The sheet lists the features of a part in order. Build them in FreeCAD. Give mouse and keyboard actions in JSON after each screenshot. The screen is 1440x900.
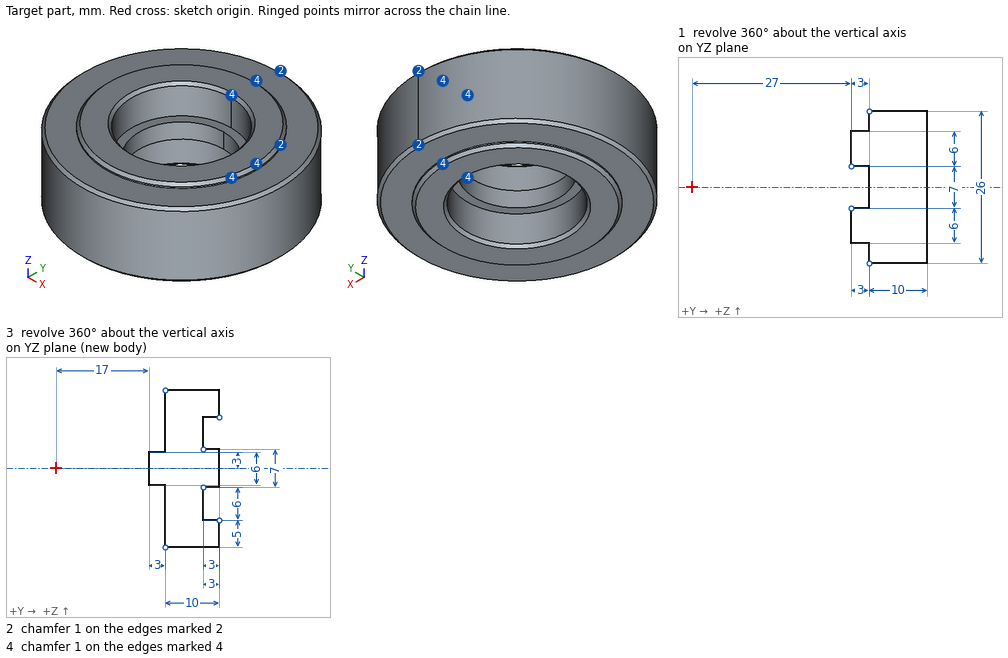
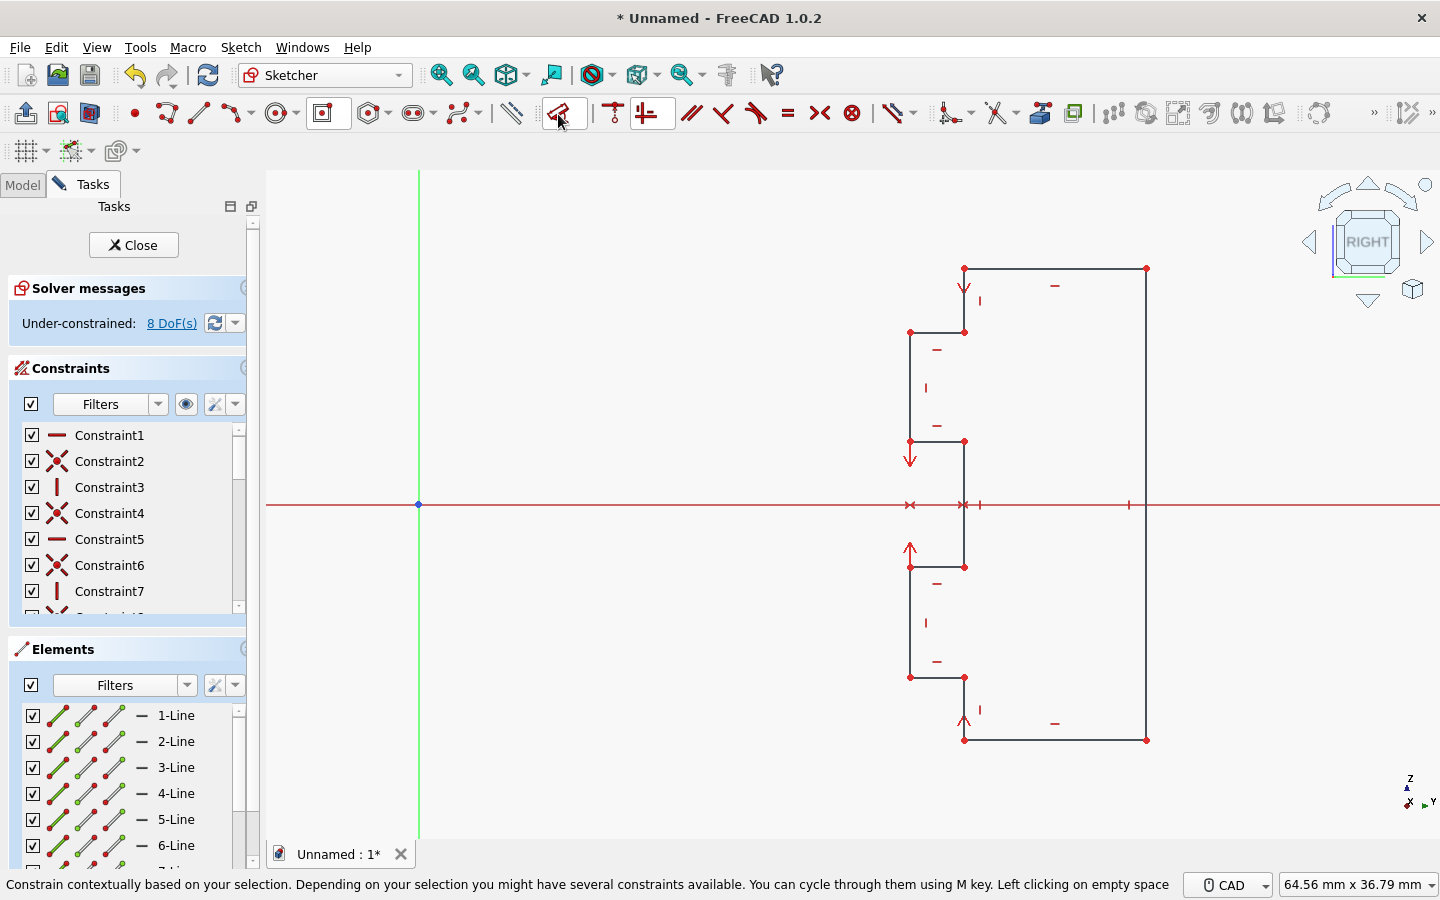
{"action": "left_click", "coordinate": [926, 442]}
{"action": "left_click", "coordinate": [937, 408]}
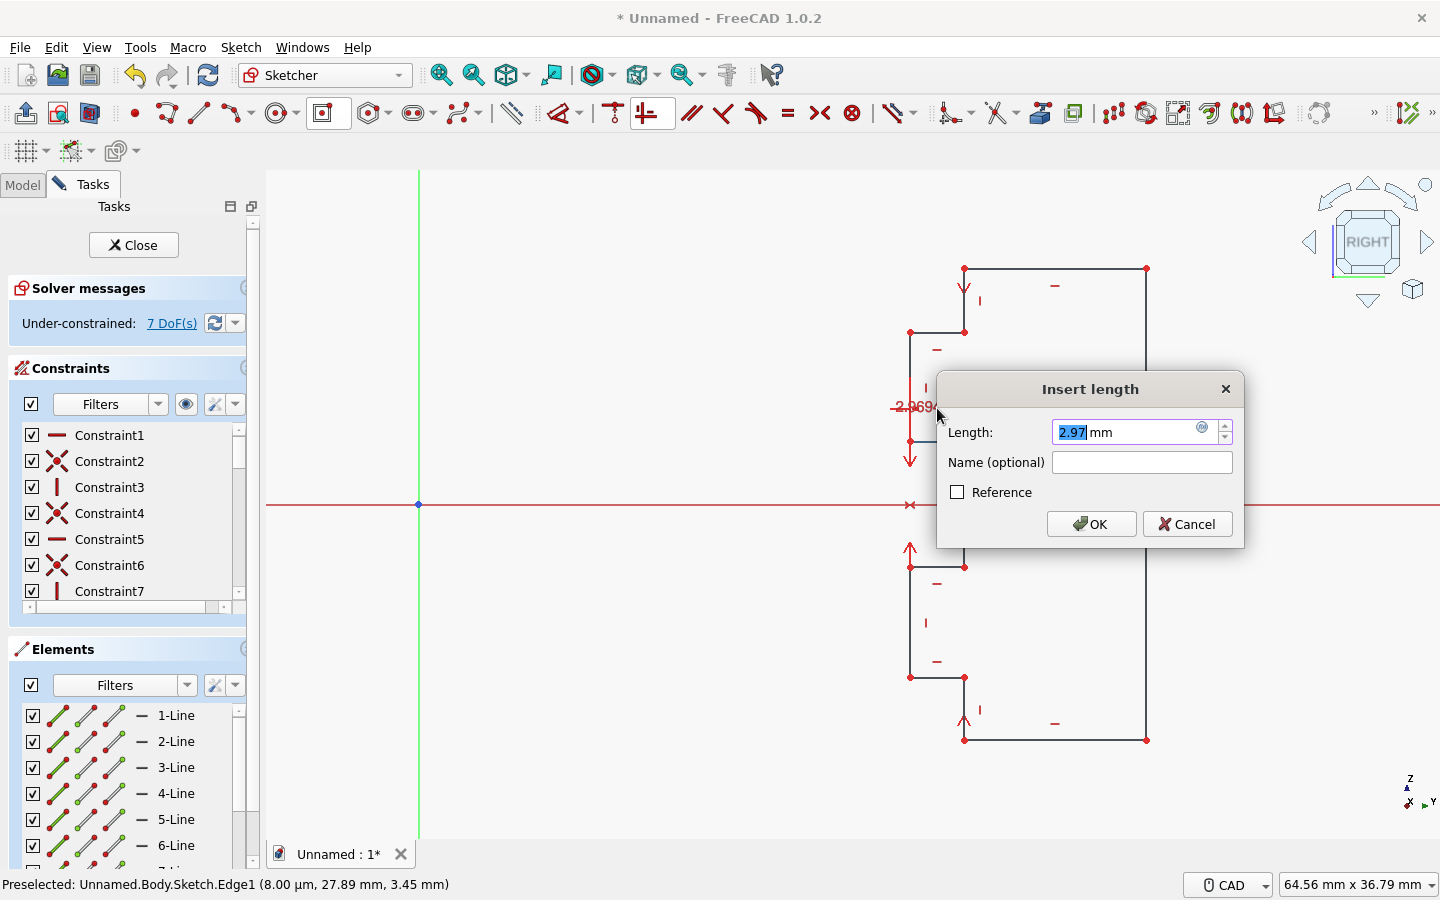
{"action": "type", "text": "3"}
{"action": "key", "text": "Return"}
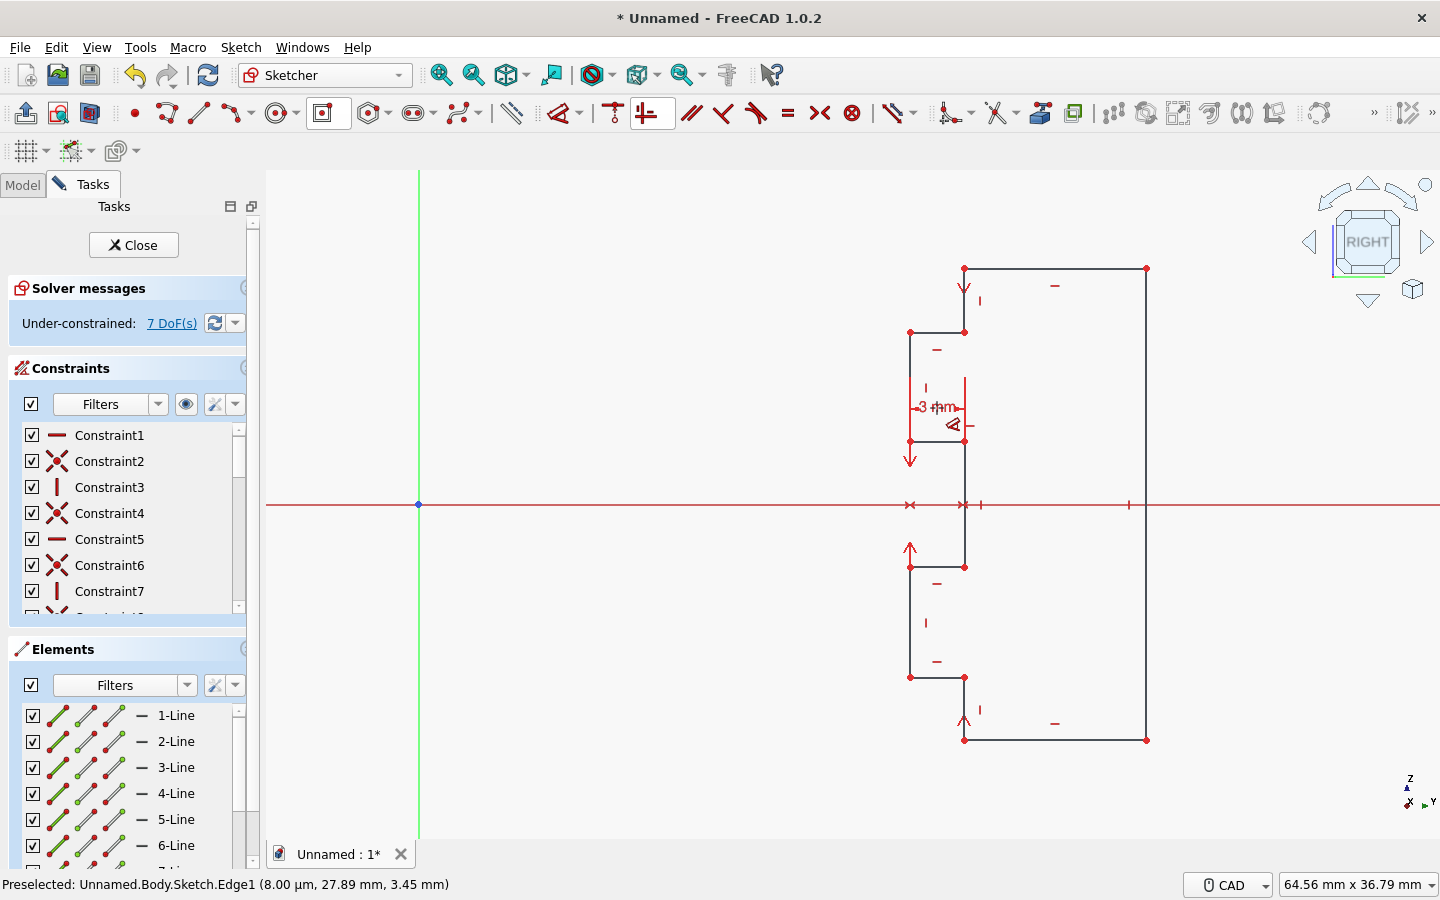
{"action": "left_click", "coordinate": [965, 479]}
{"action": "left_click", "coordinate": [999, 476]}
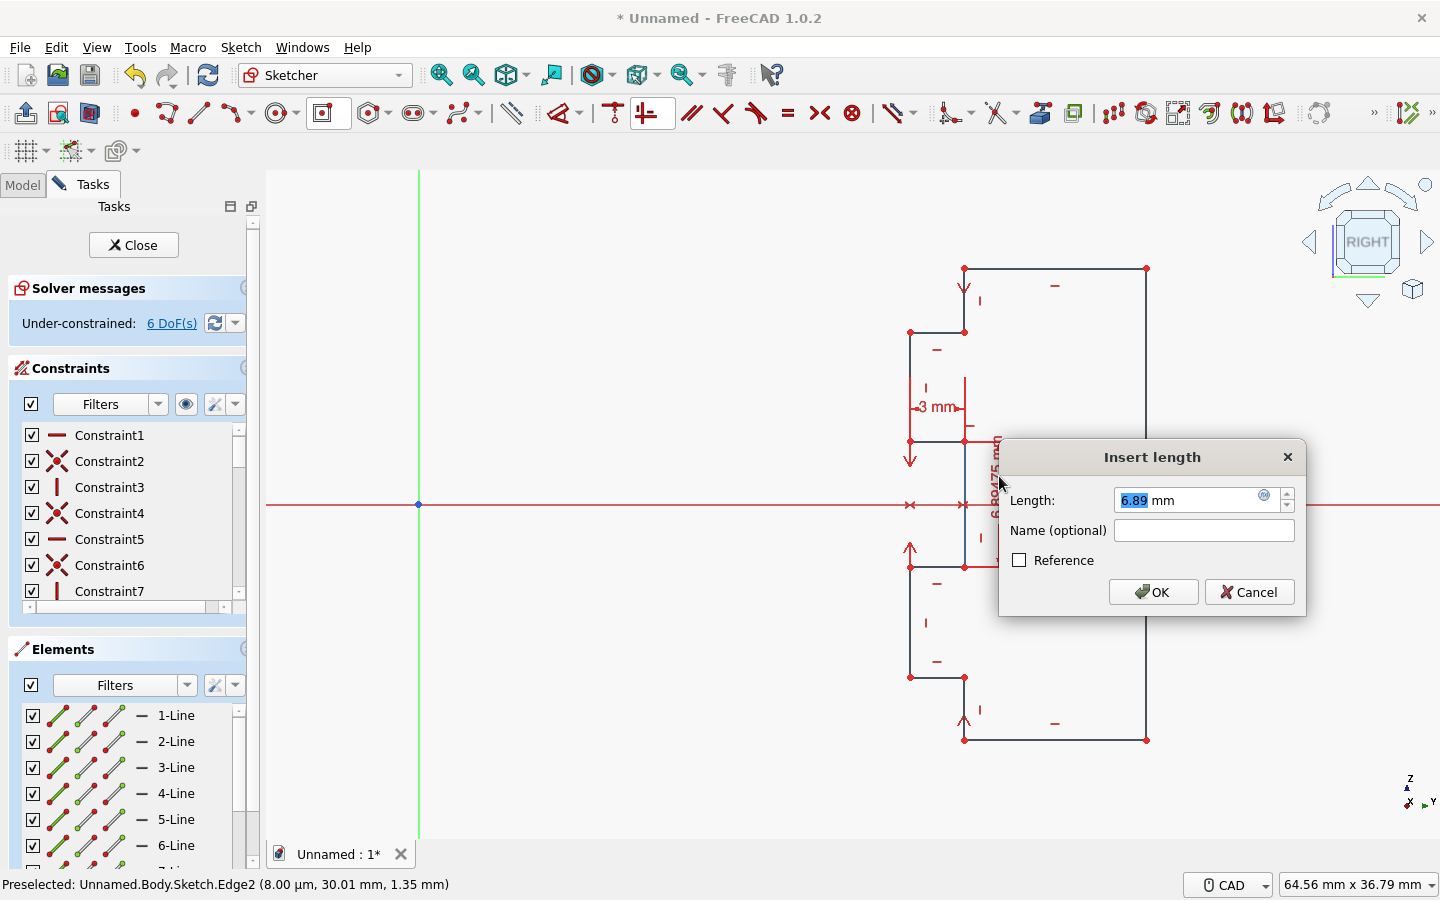
{"action": "type", "text": "7"}
{"action": "key", "text": "Return"}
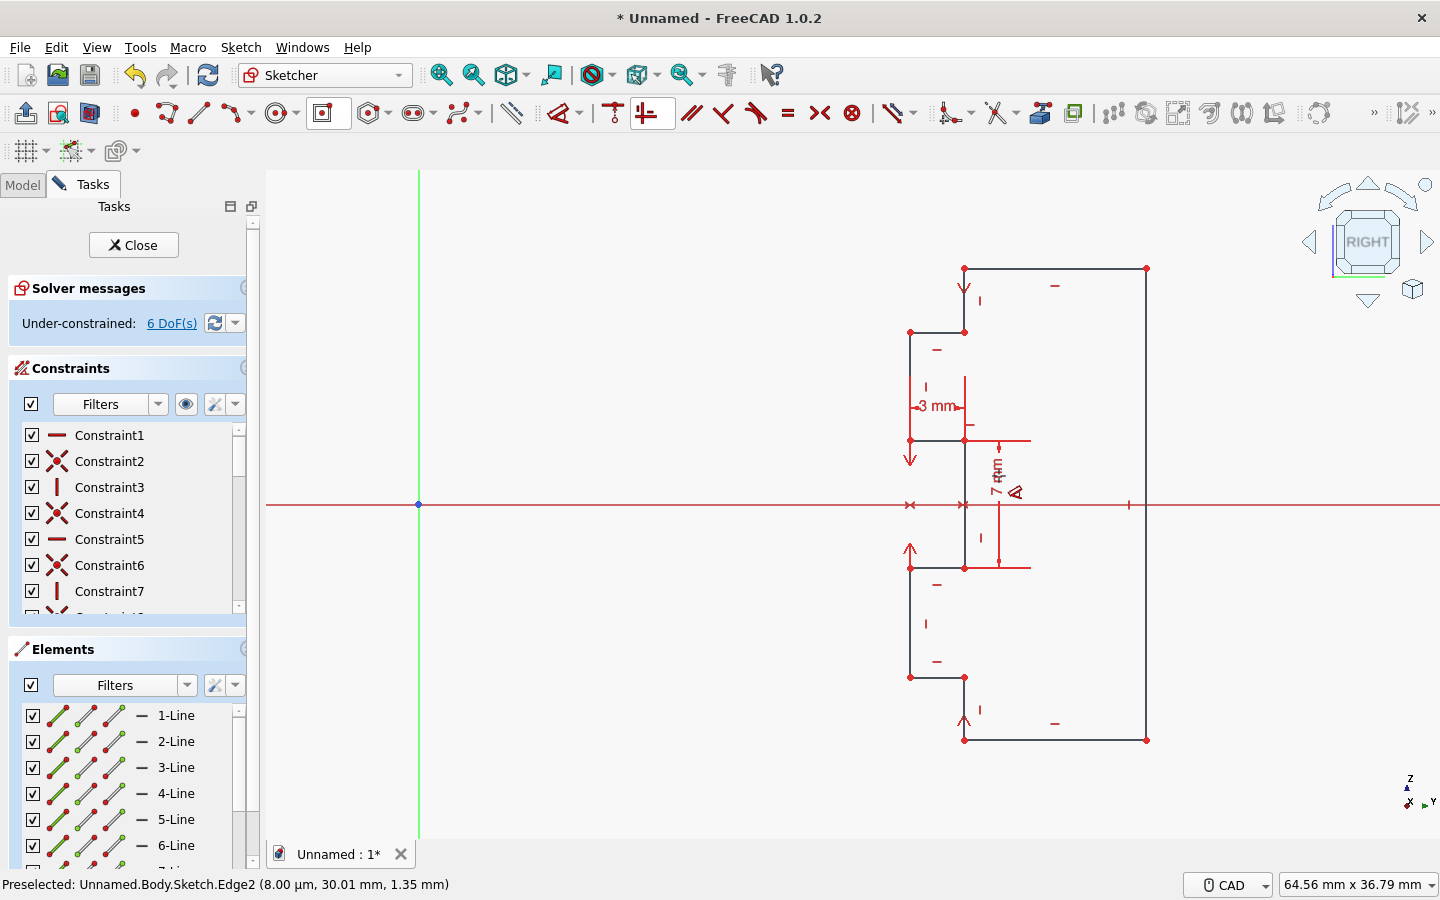
{"action": "left_click", "coordinate": [910, 601]}
{"action": "left_click", "coordinate": [944, 623]}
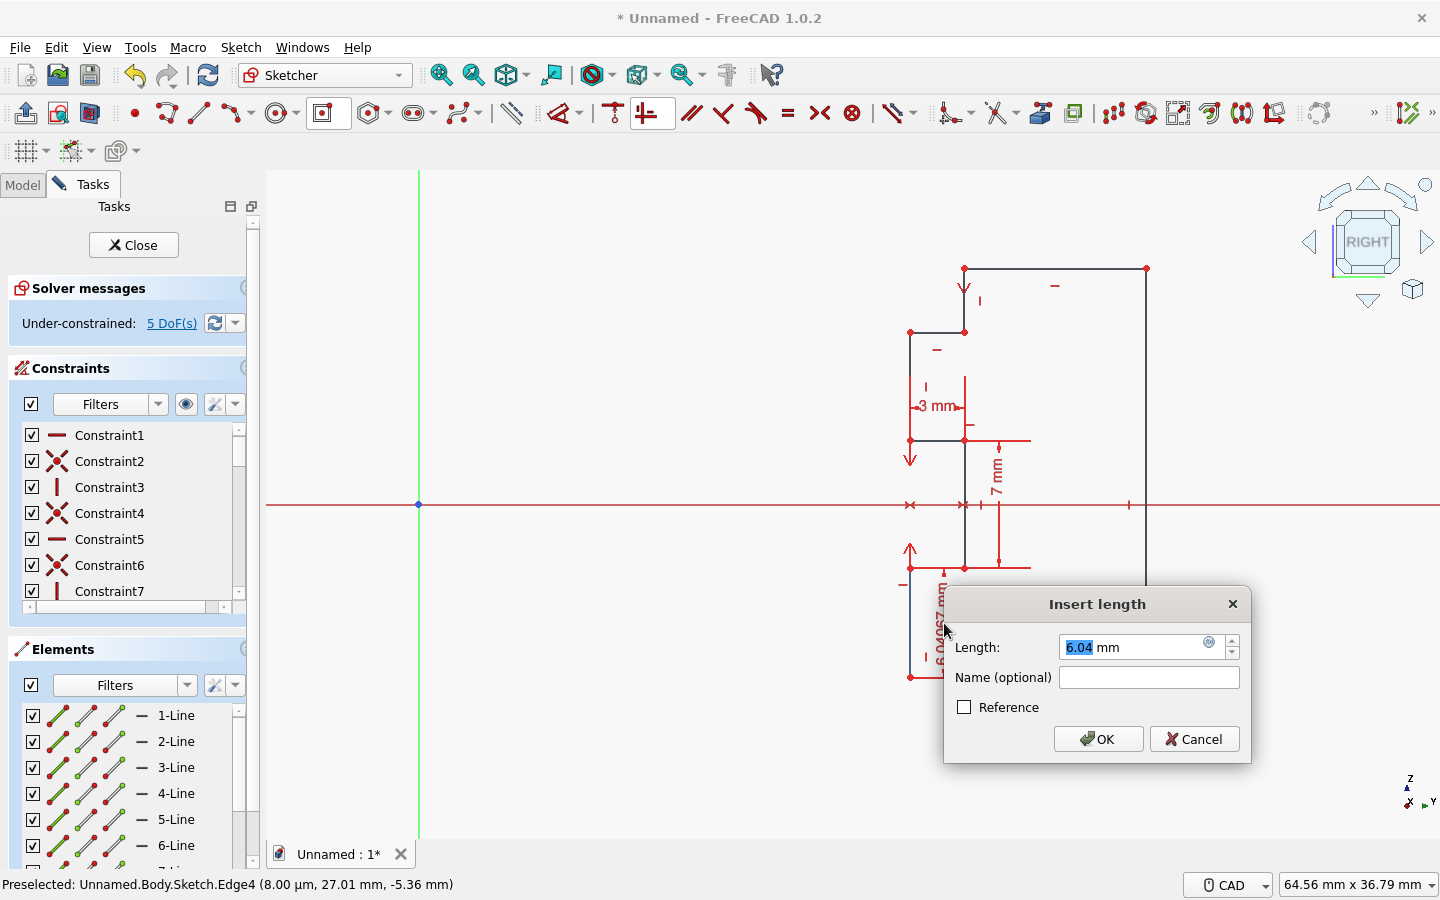
{"action": "type", "text": "6"}
{"action": "key", "text": "Return"}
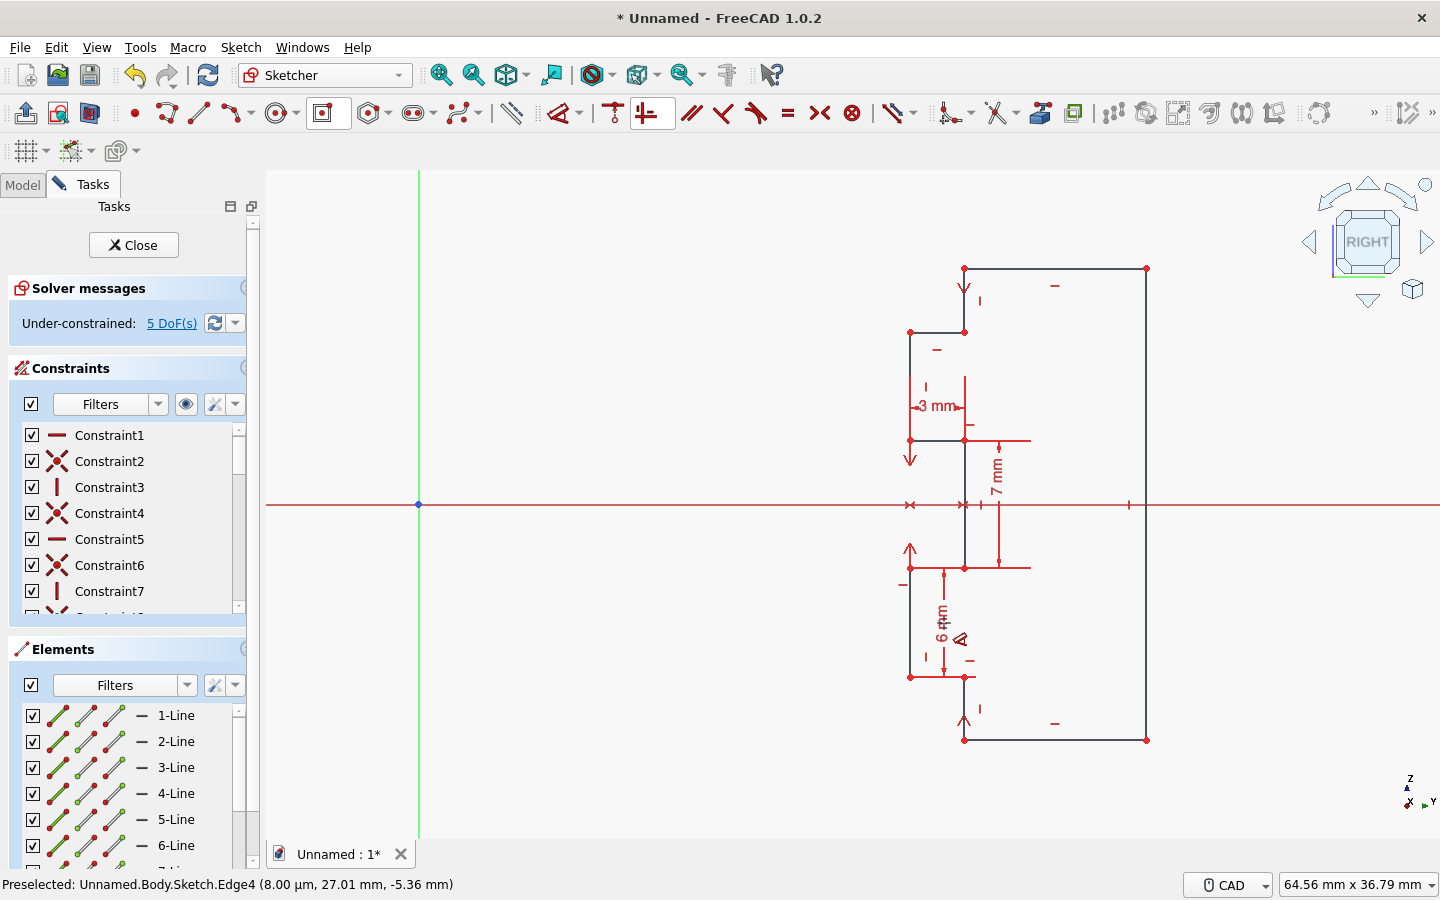
{"action": "left_click", "coordinate": [926, 677]}
{"action": "left_click", "coordinate": [937, 711]}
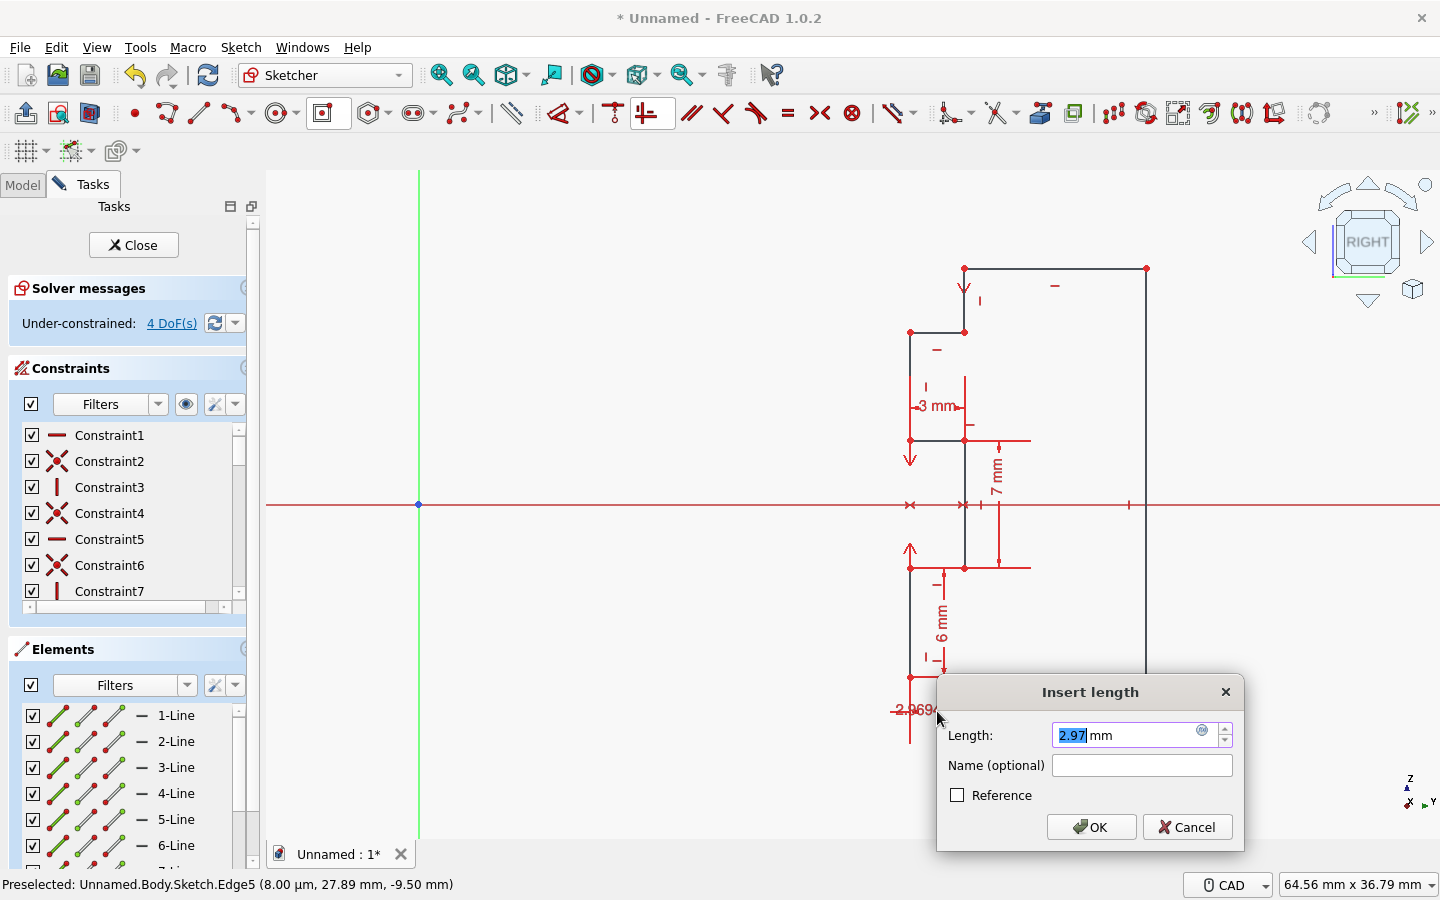
{"action": "type", "text": "3"}
{"action": "key", "text": "Return"}